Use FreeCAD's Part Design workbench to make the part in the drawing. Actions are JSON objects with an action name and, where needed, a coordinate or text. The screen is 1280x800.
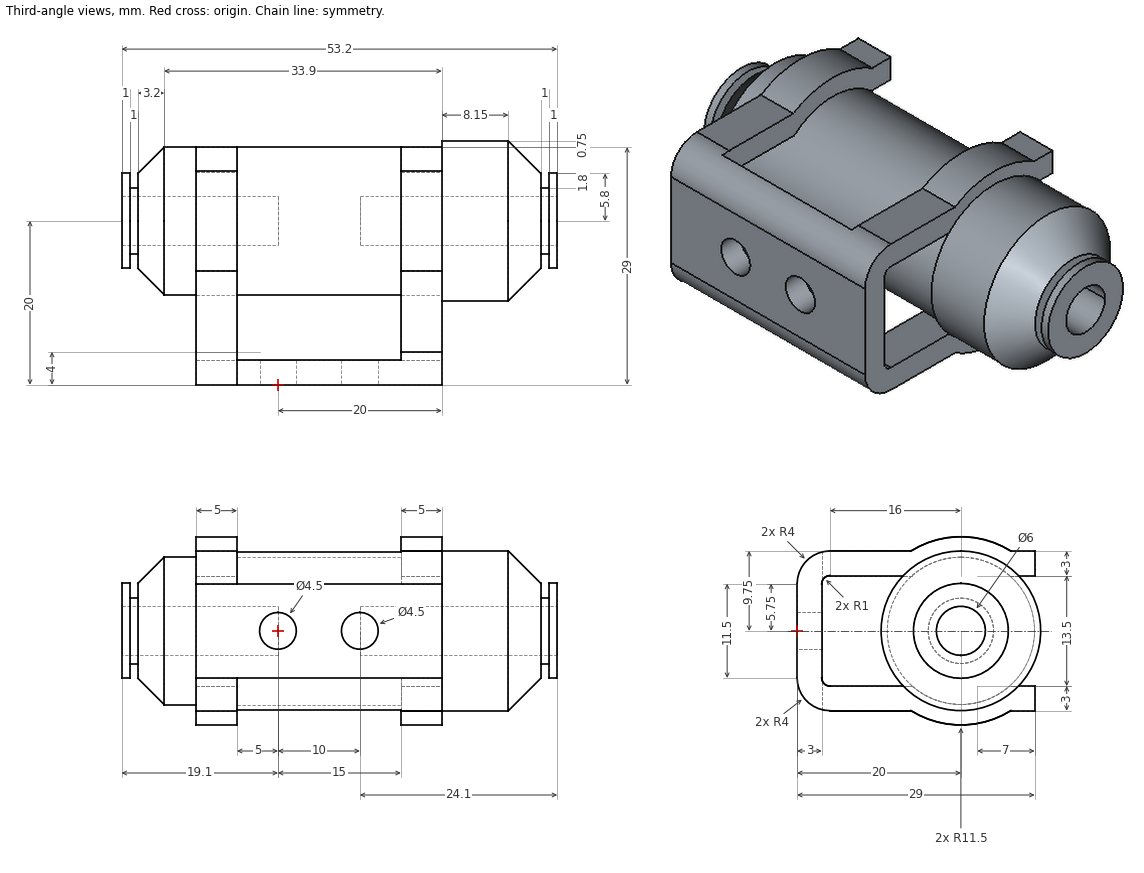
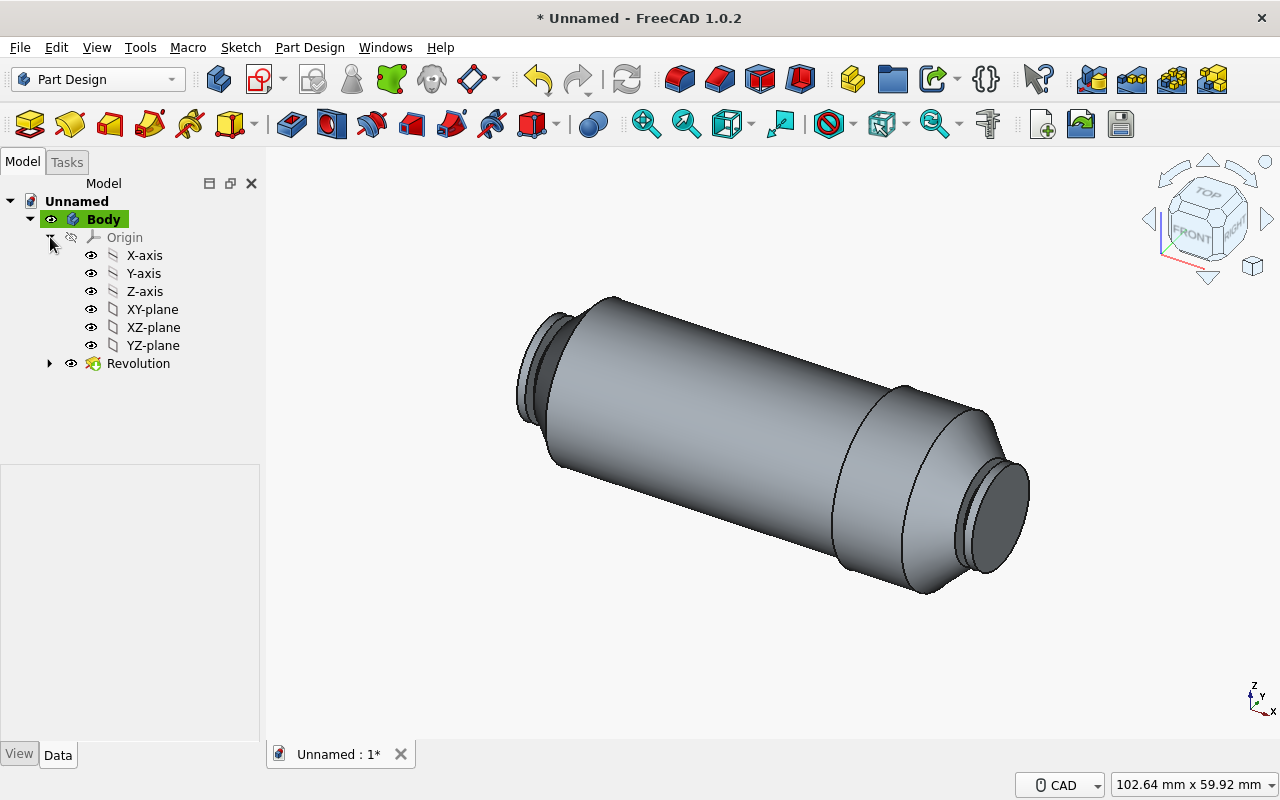
{"action": "left_click", "coordinate": [136, 345]}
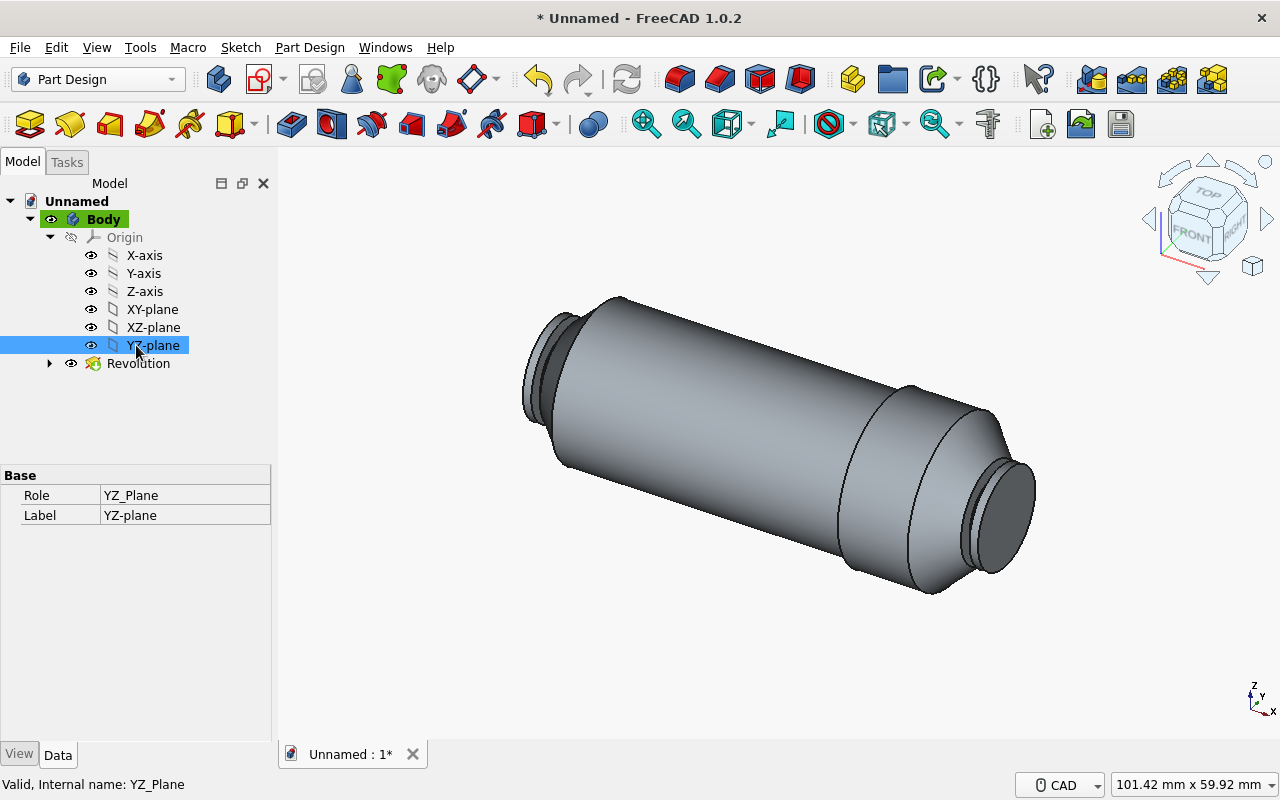
{"action": "left_click", "coordinate": [472, 80]}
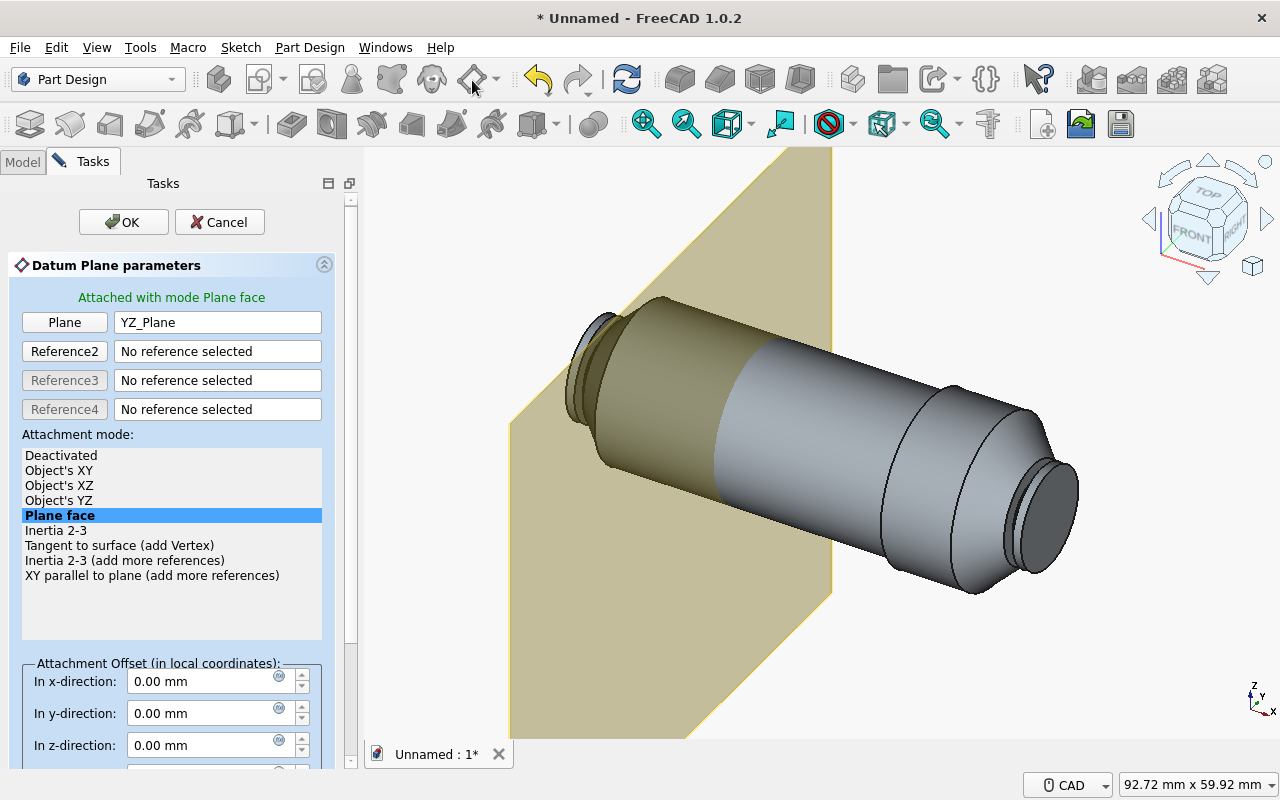
{"action": "triple_click", "coordinate": [210, 745]}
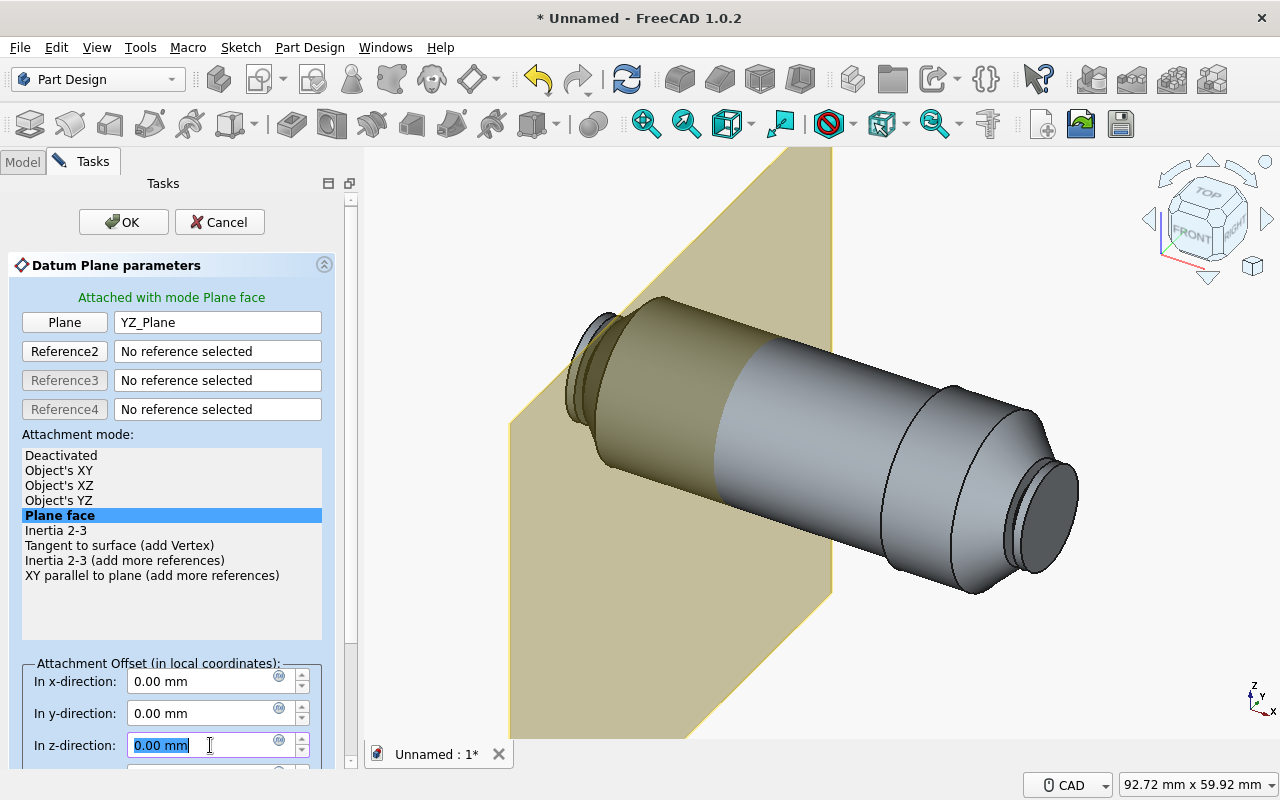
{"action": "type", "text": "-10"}
{"action": "key", "text": "Tab"}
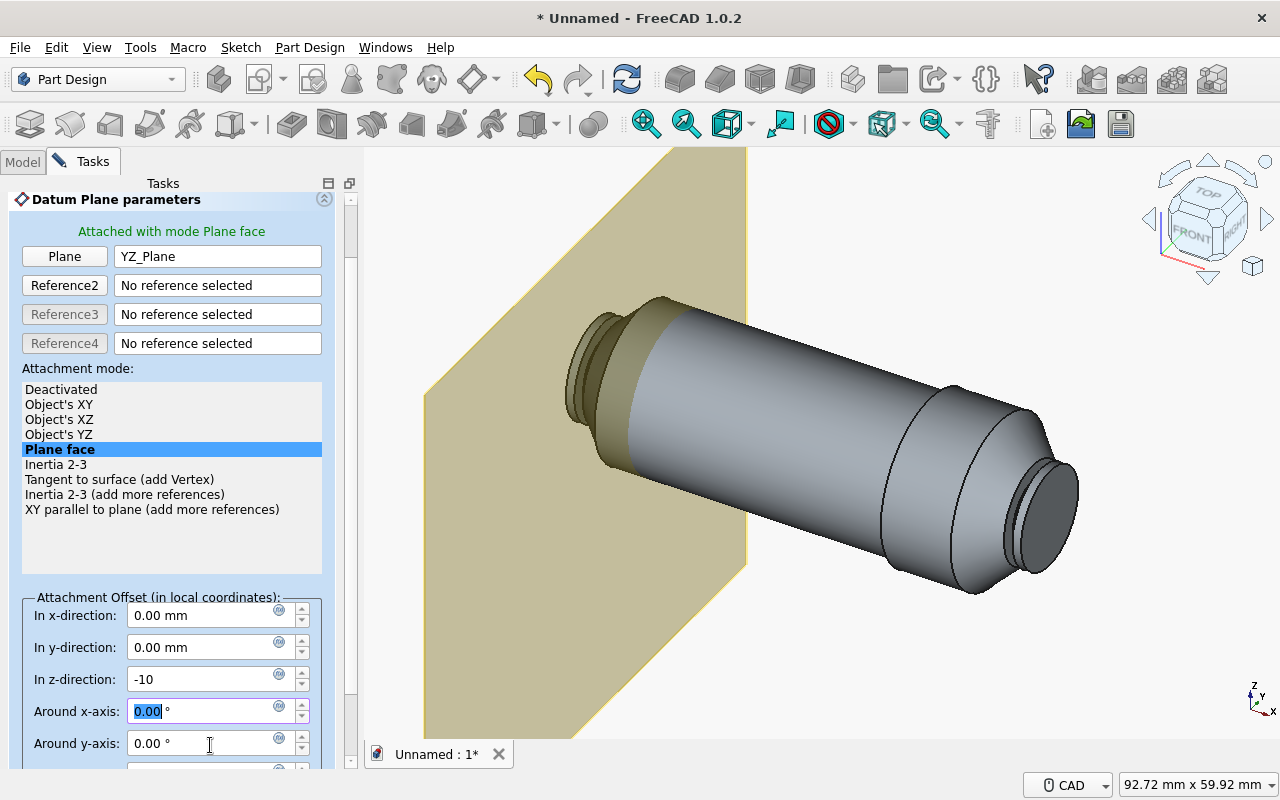
{"action": "scroll", "coordinate": [351, 480], "scroll_direction": "up", "scroll_amount": 2}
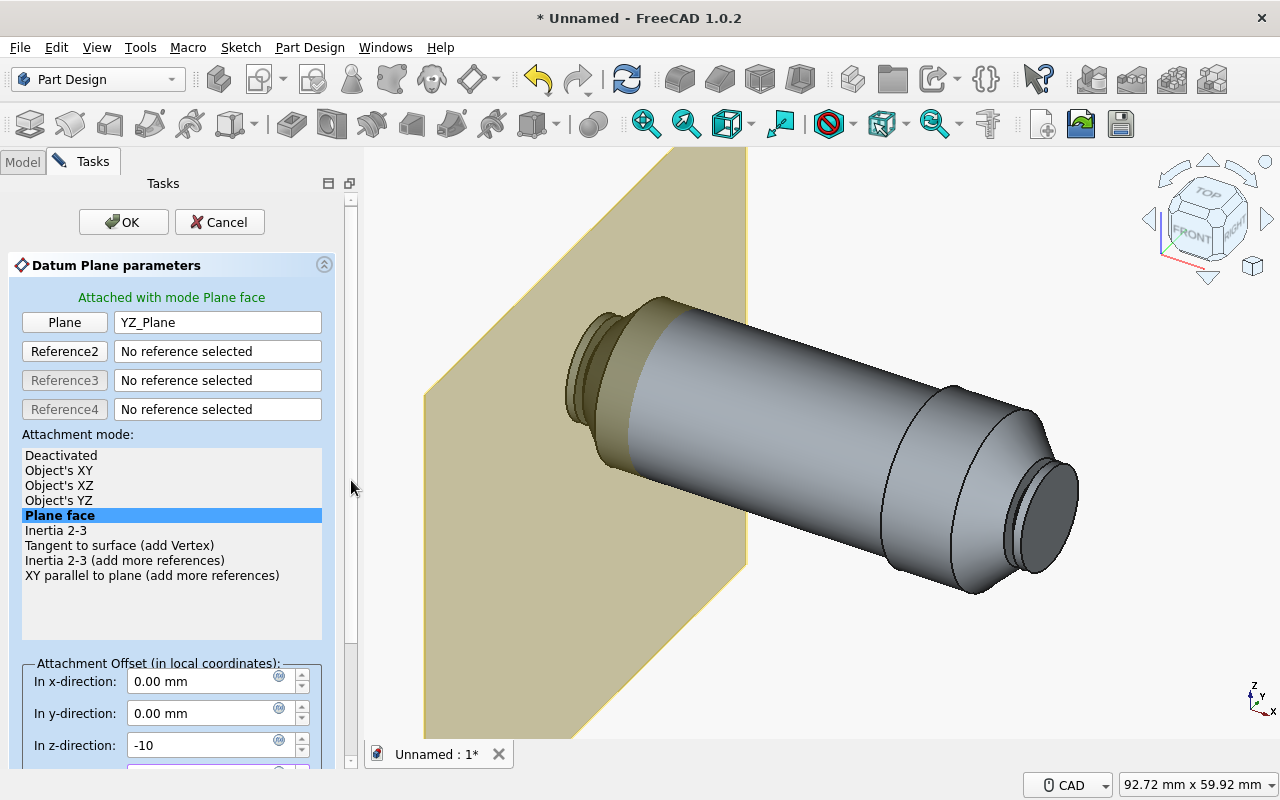
{"action": "left_click", "coordinate": [124, 222]}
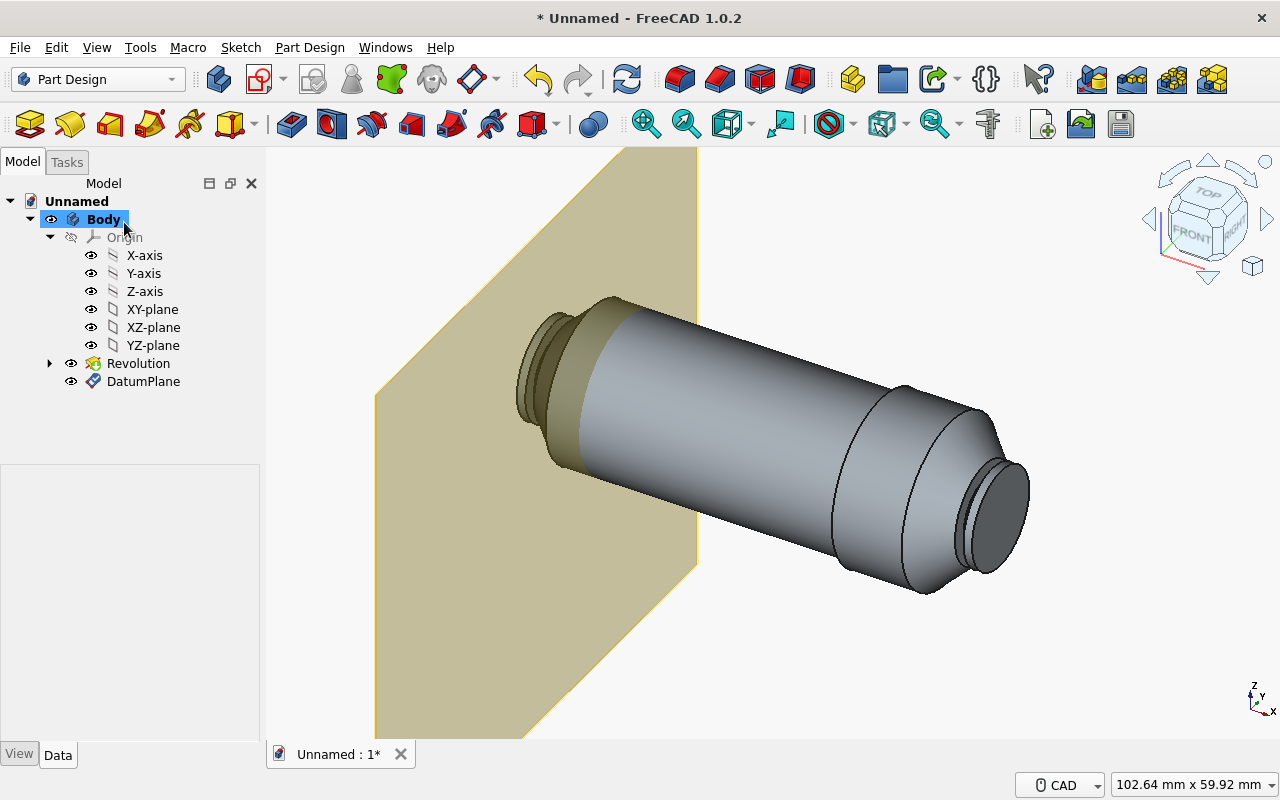
{"action": "left_click", "coordinate": [116, 381]}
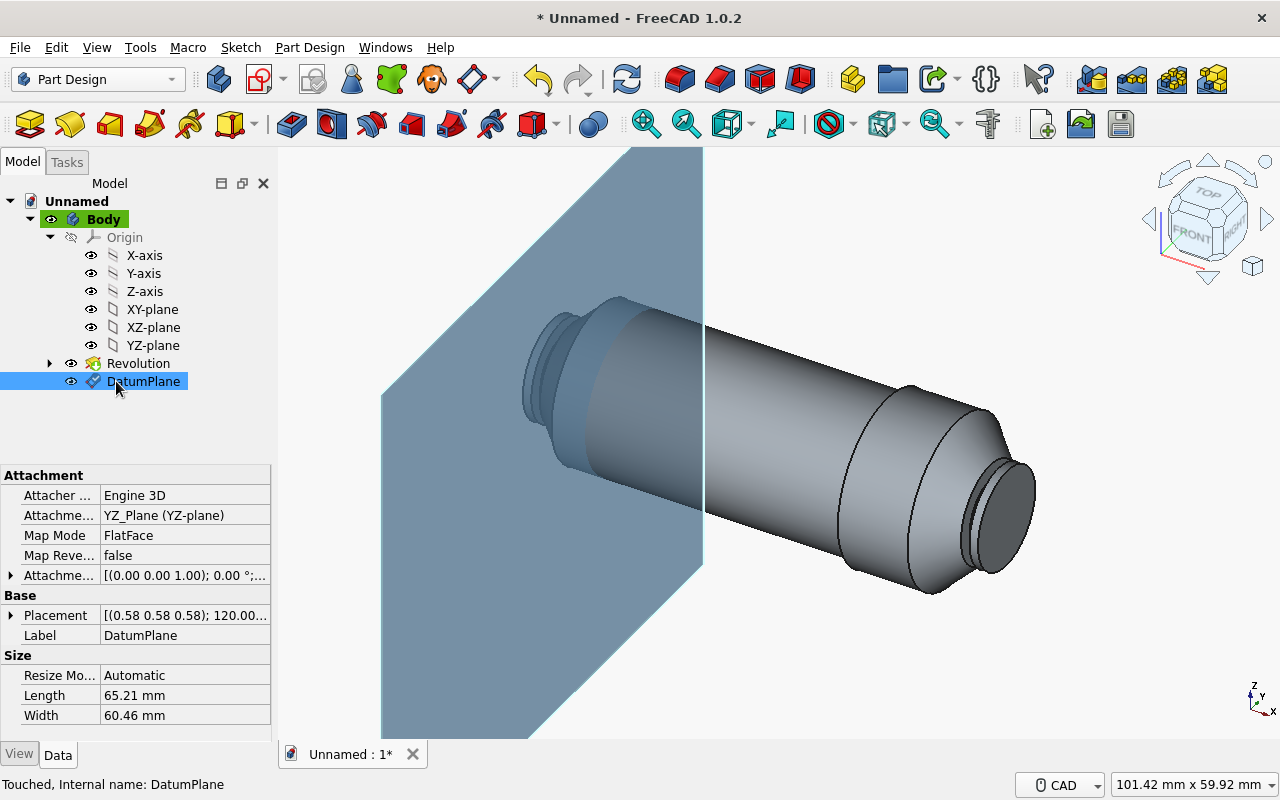
{"action": "left_click", "coordinate": [260, 80]}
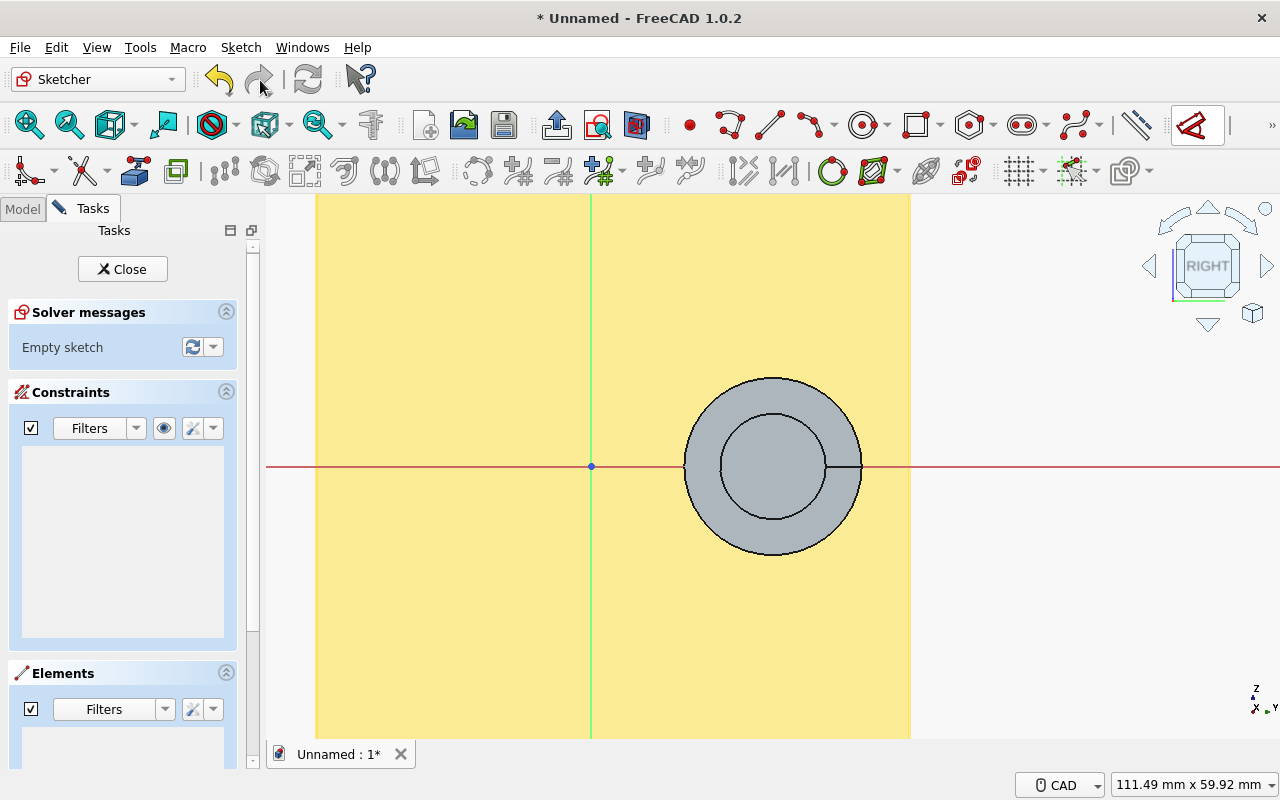
{"action": "left_click", "coordinate": [638, 126]}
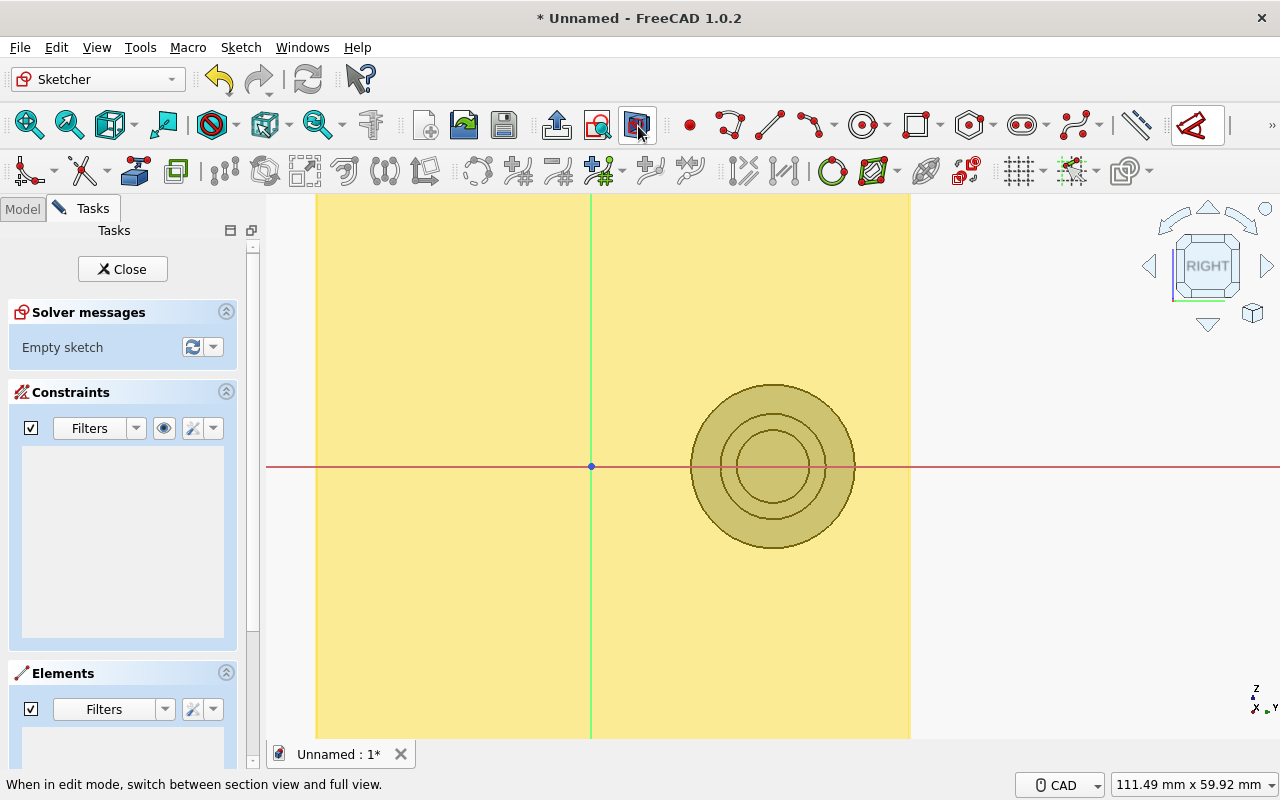
{"action": "scroll", "coordinate": [745, 466], "scroll_direction": "up", "scroll_amount": 3}